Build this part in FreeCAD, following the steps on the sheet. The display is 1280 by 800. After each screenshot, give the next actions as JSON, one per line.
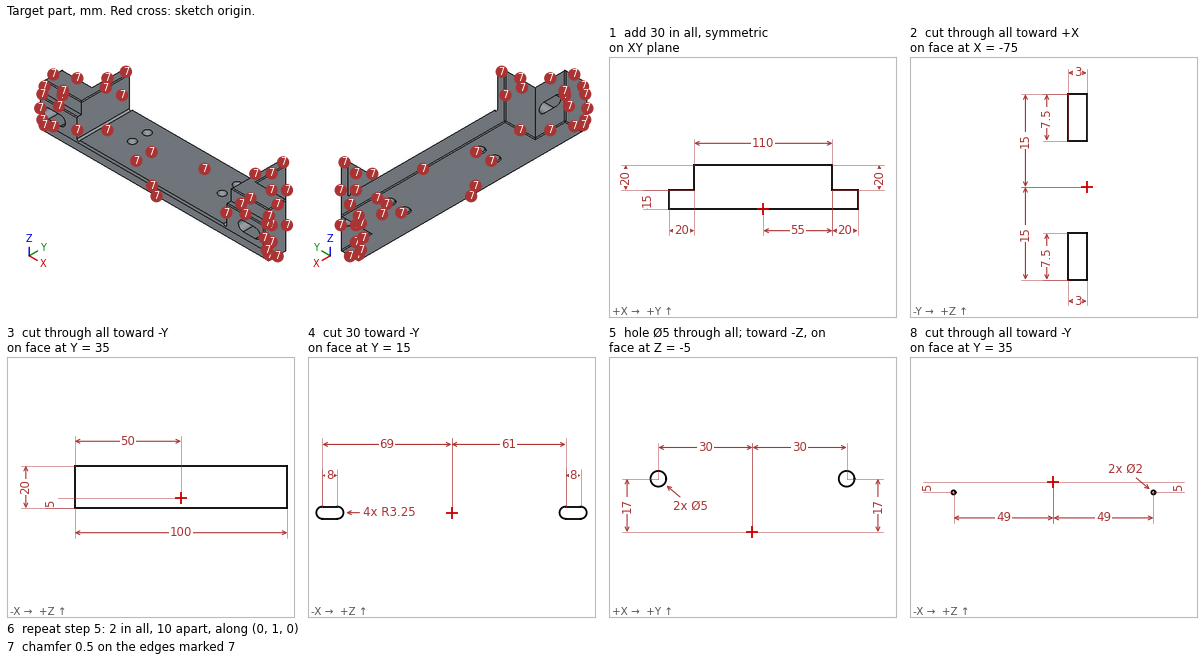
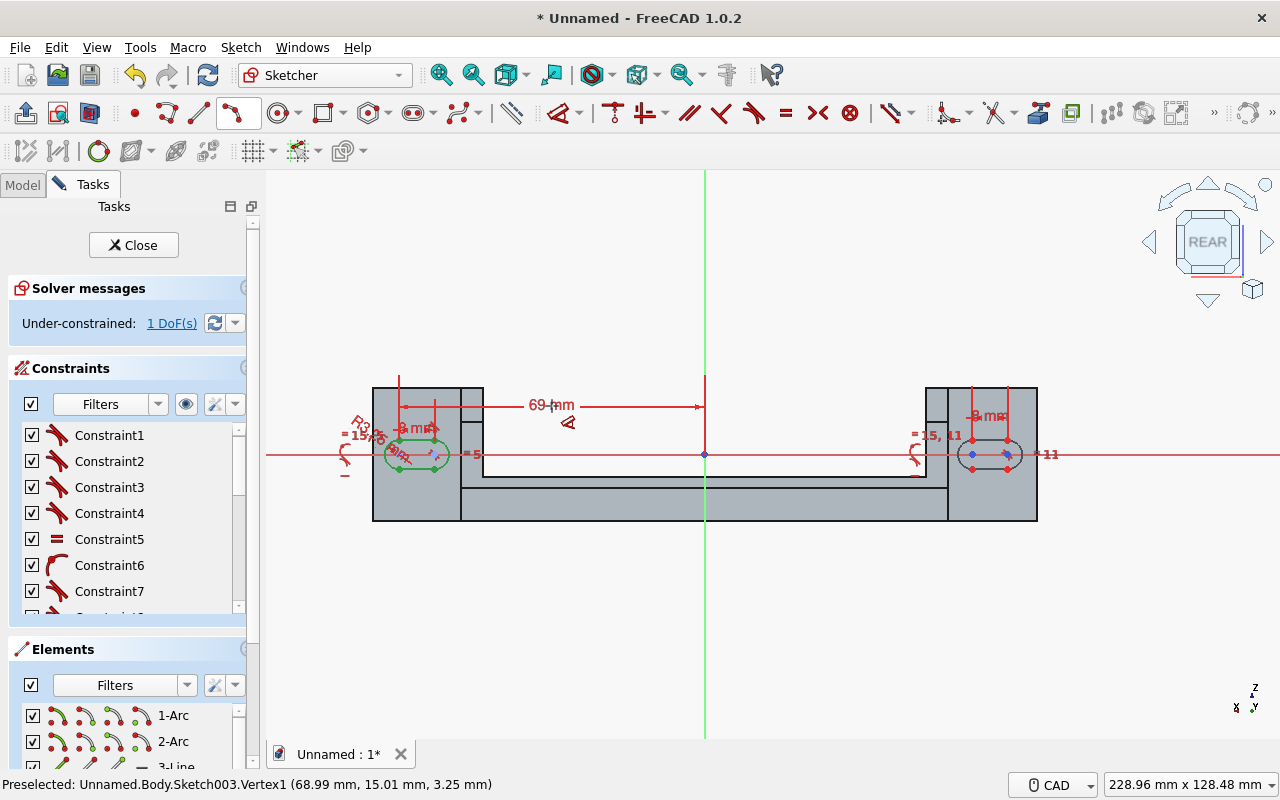
{"action": "left_click", "coordinate": [972, 440]}
{"action": "left_click", "coordinate": [839, 406]}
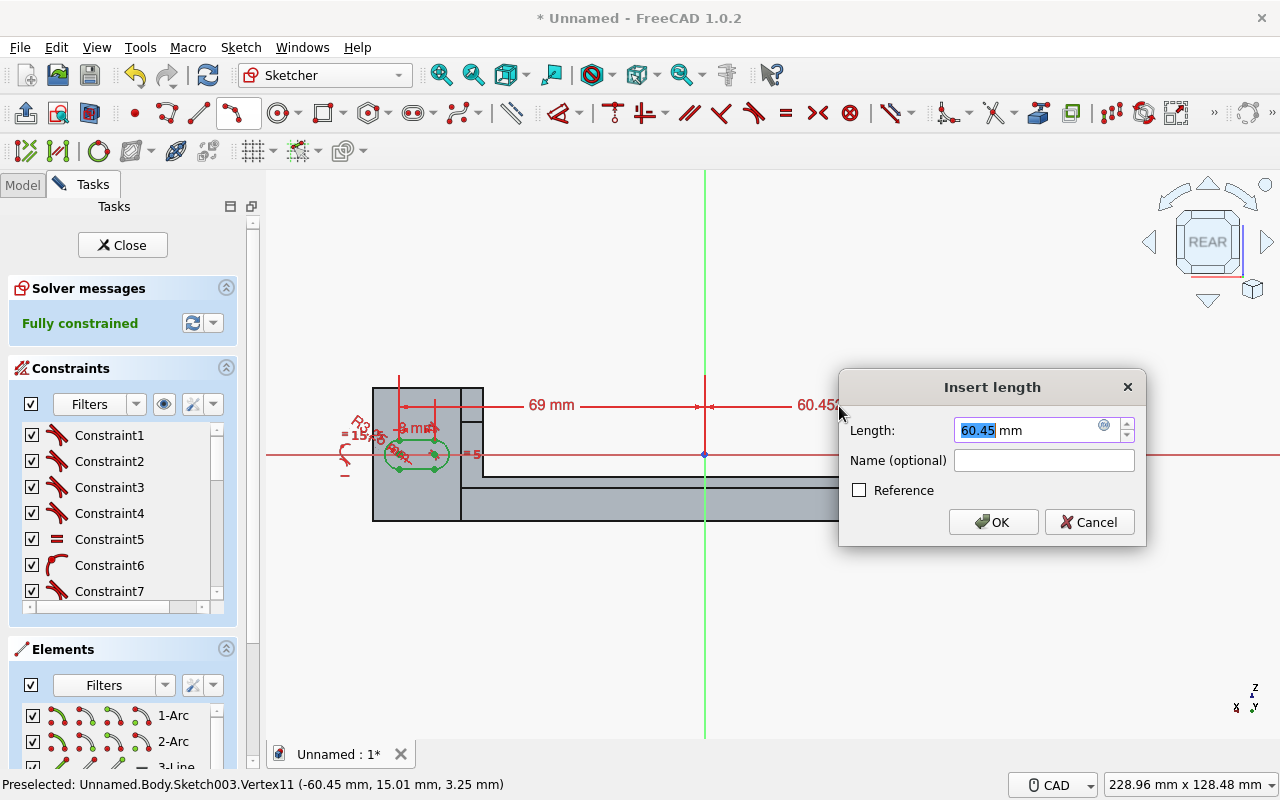
{"action": "type", "text": "61"}
{"action": "key", "text": "Return"}
{"action": "key", "text": "Escape"}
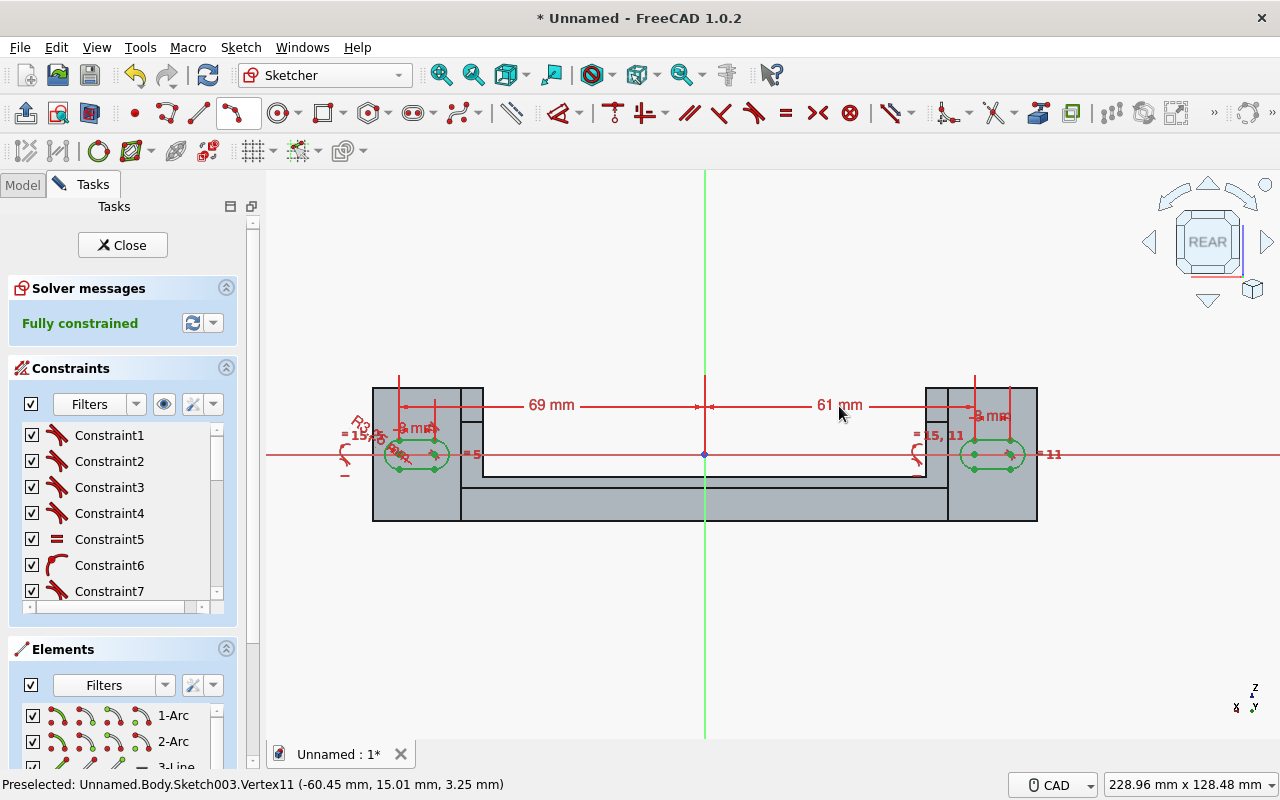
{"action": "left_click", "coordinate": [123, 245]}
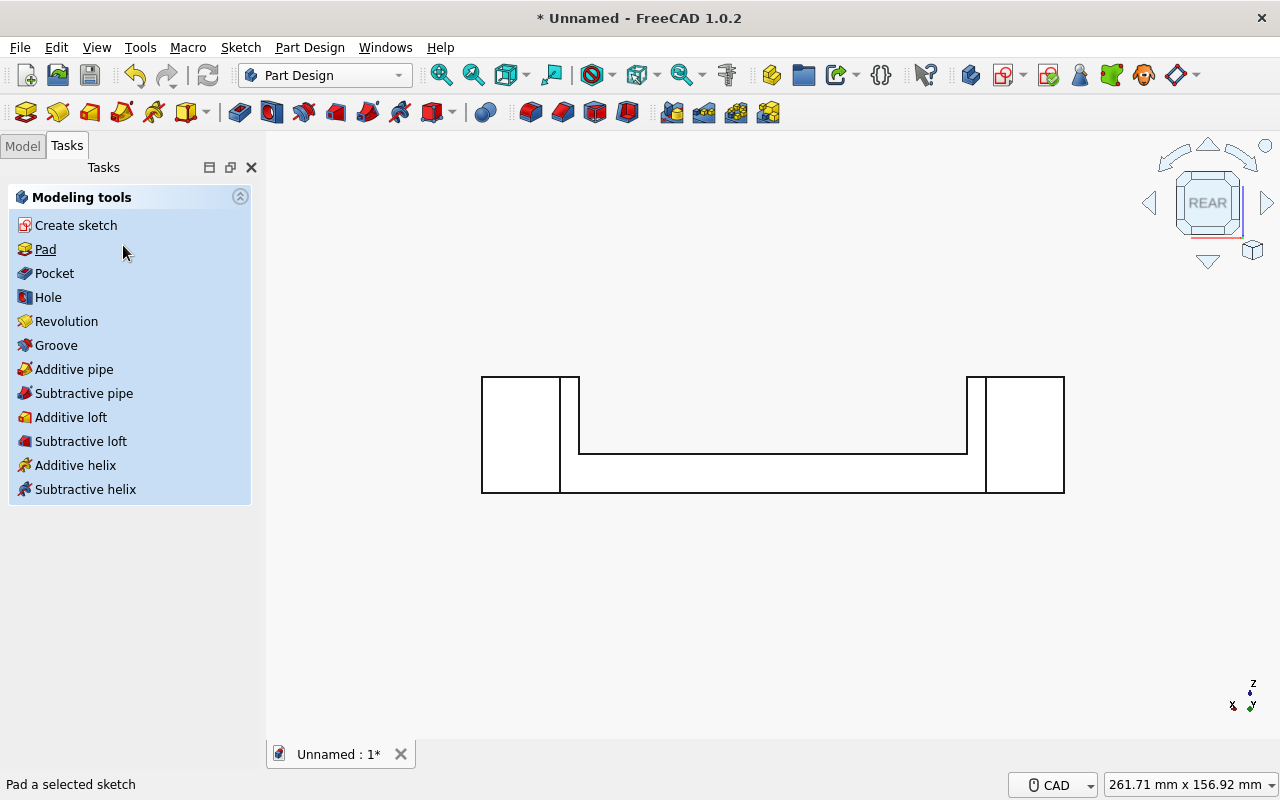
{"action": "left_click", "coordinate": [240, 112]}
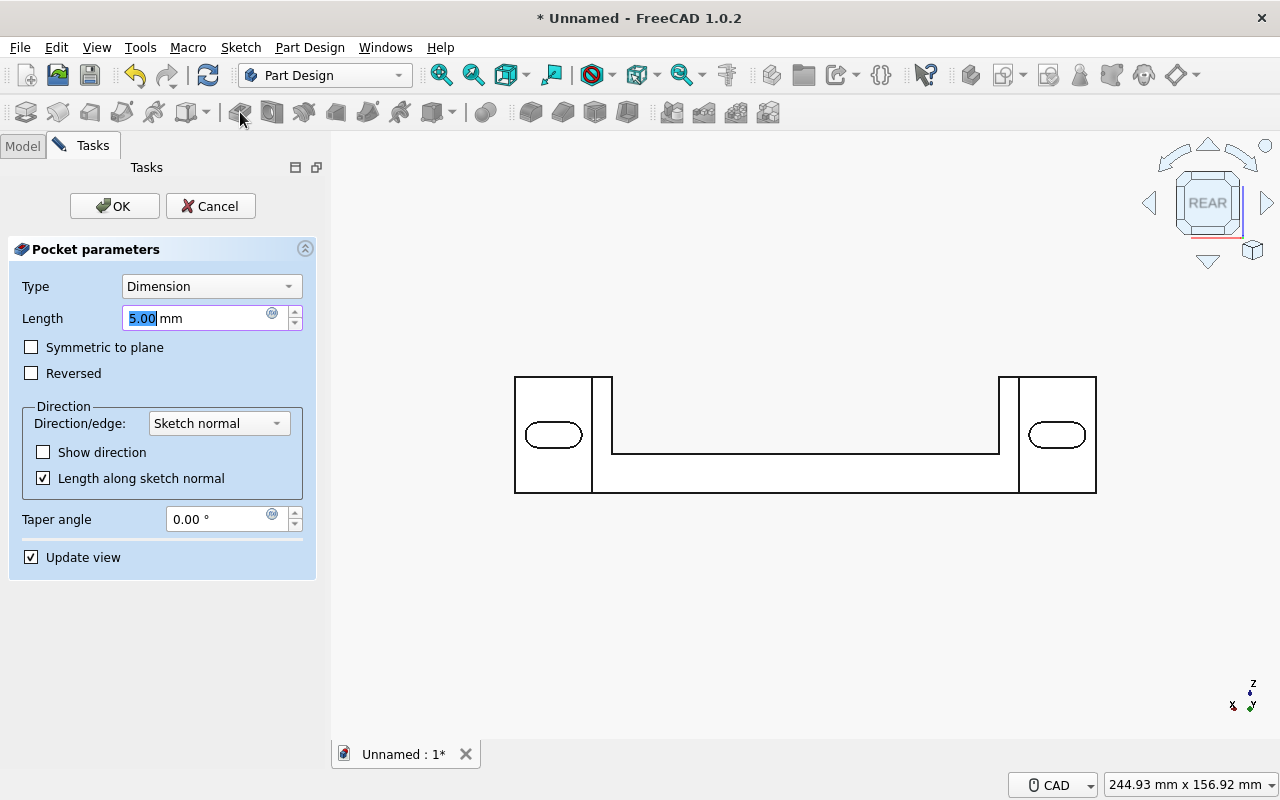
{"action": "type", "text": "30"}
{"action": "key", "text": "Tab"}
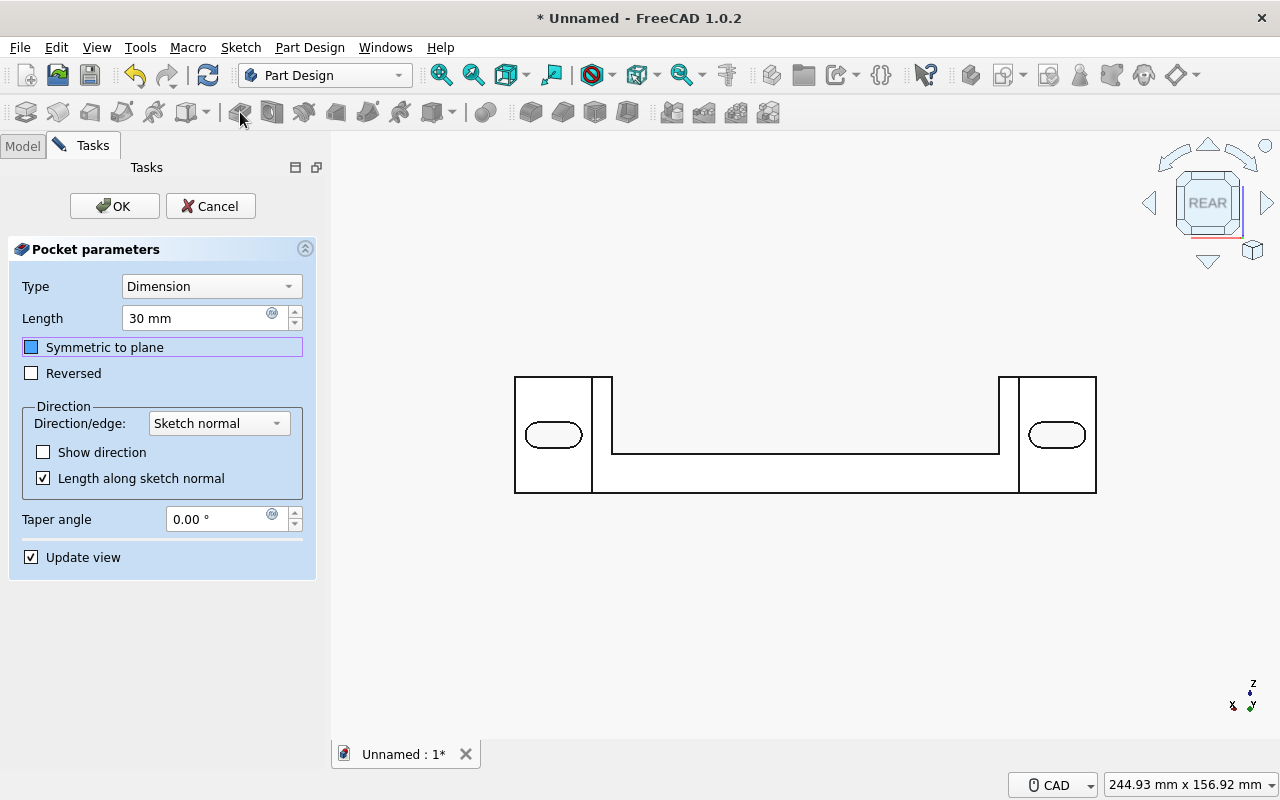
{"action": "left_click", "coordinate": [115, 206]}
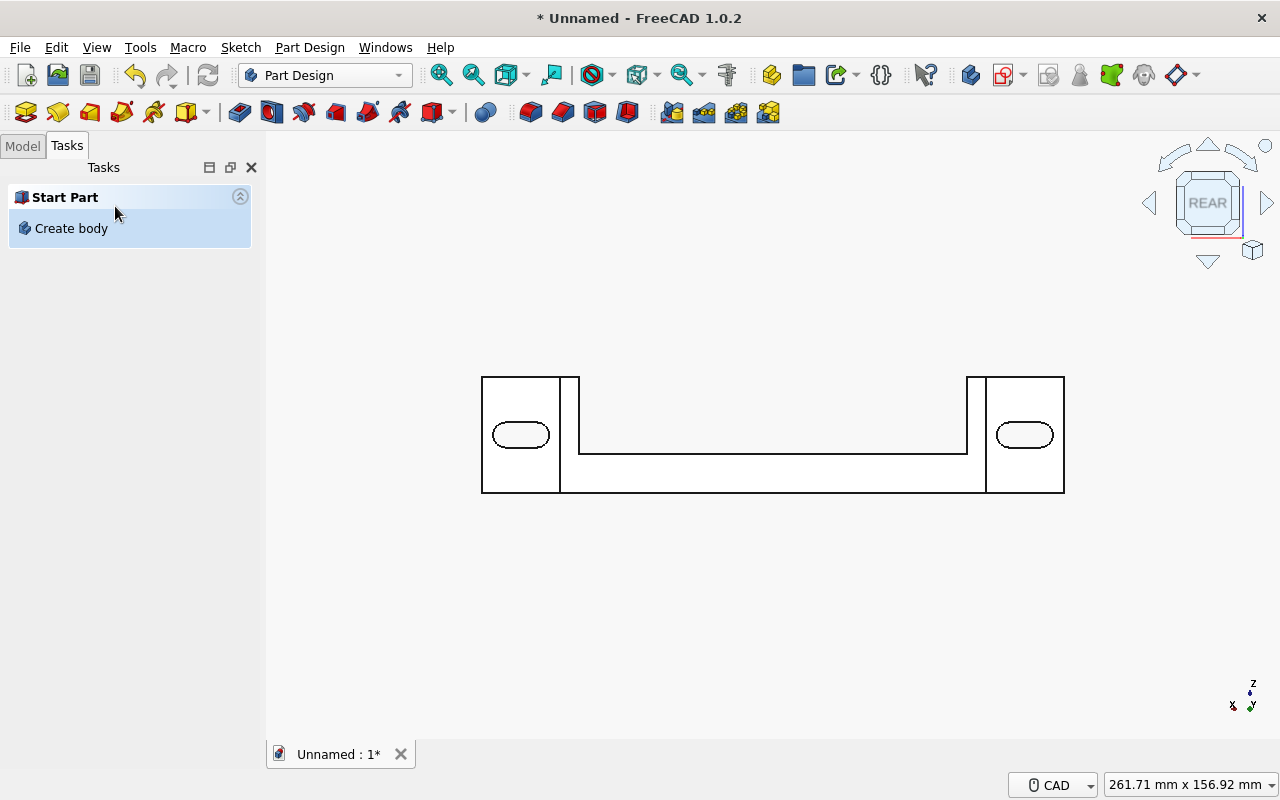
{"action": "key", "text": "0"}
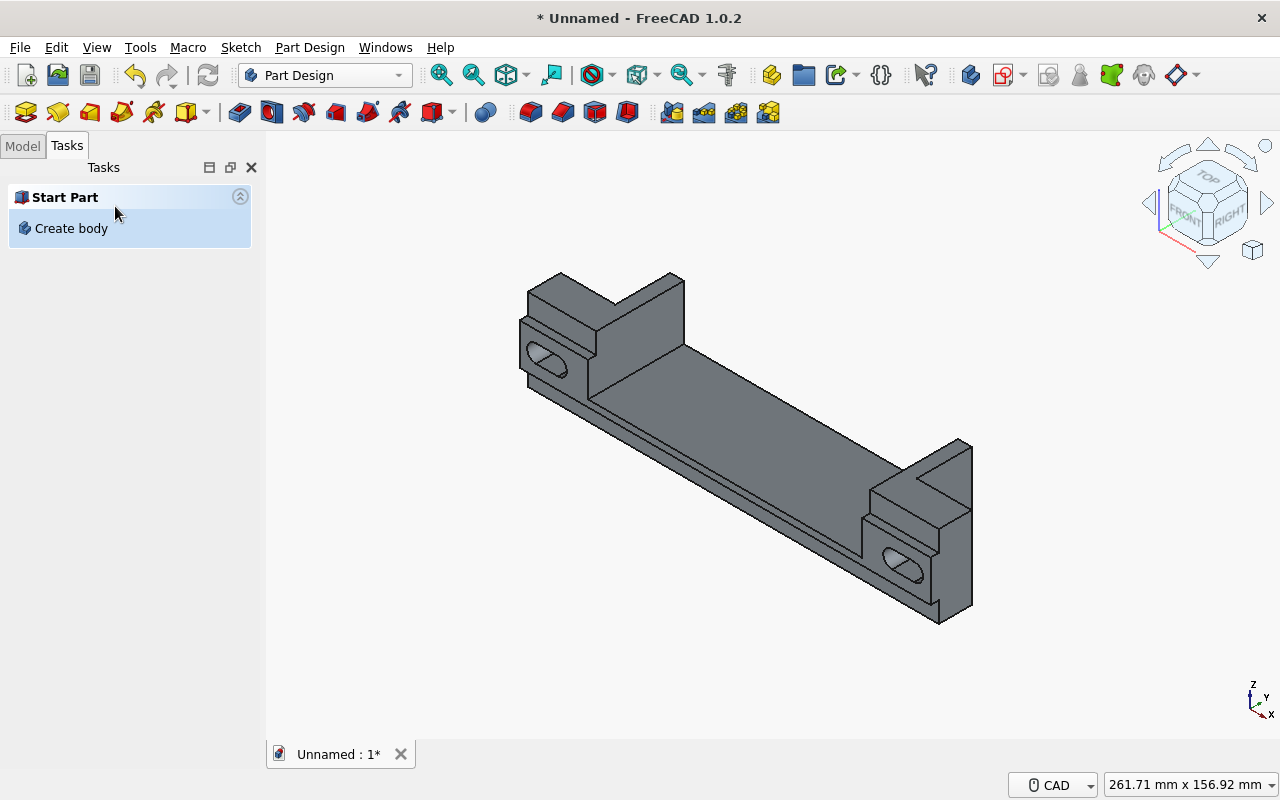
{"action": "left_click", "coordinate": [851, 495]}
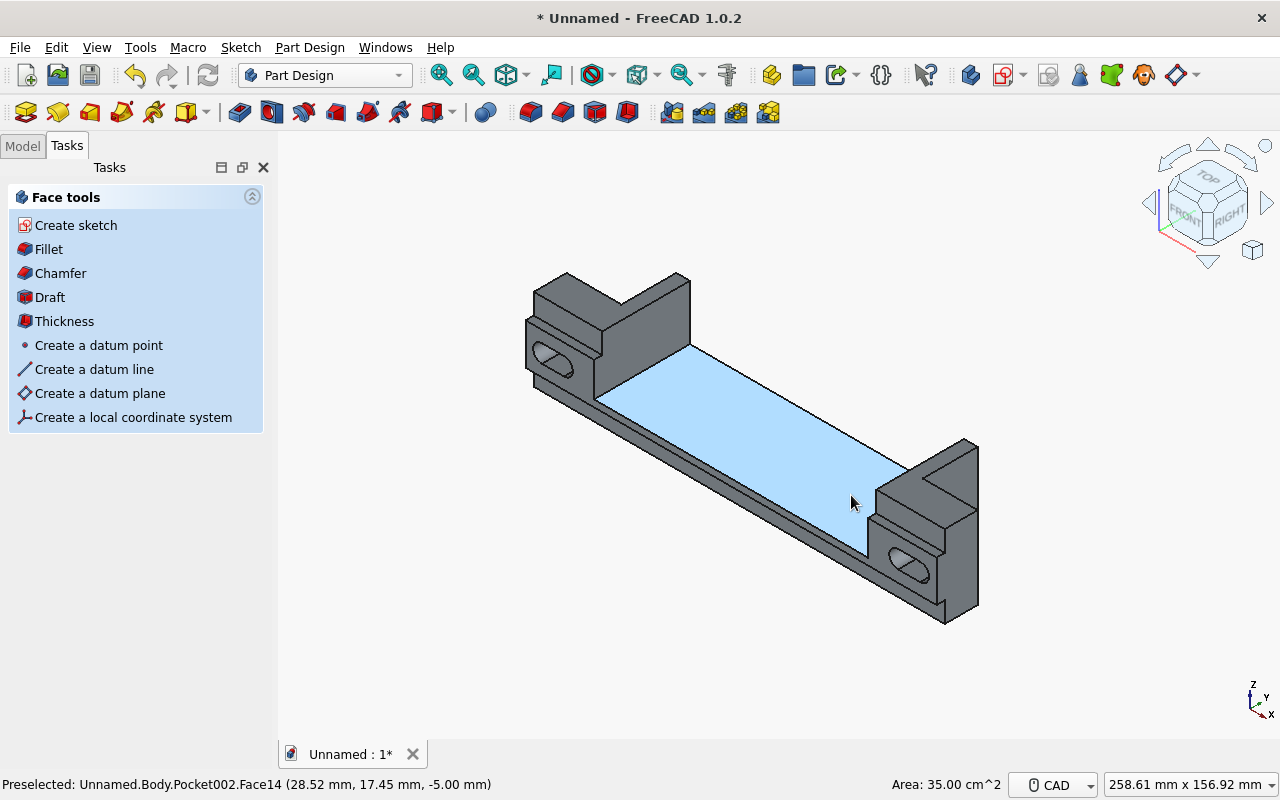
{"action": "left_click", "coordinate": [1004, 76]}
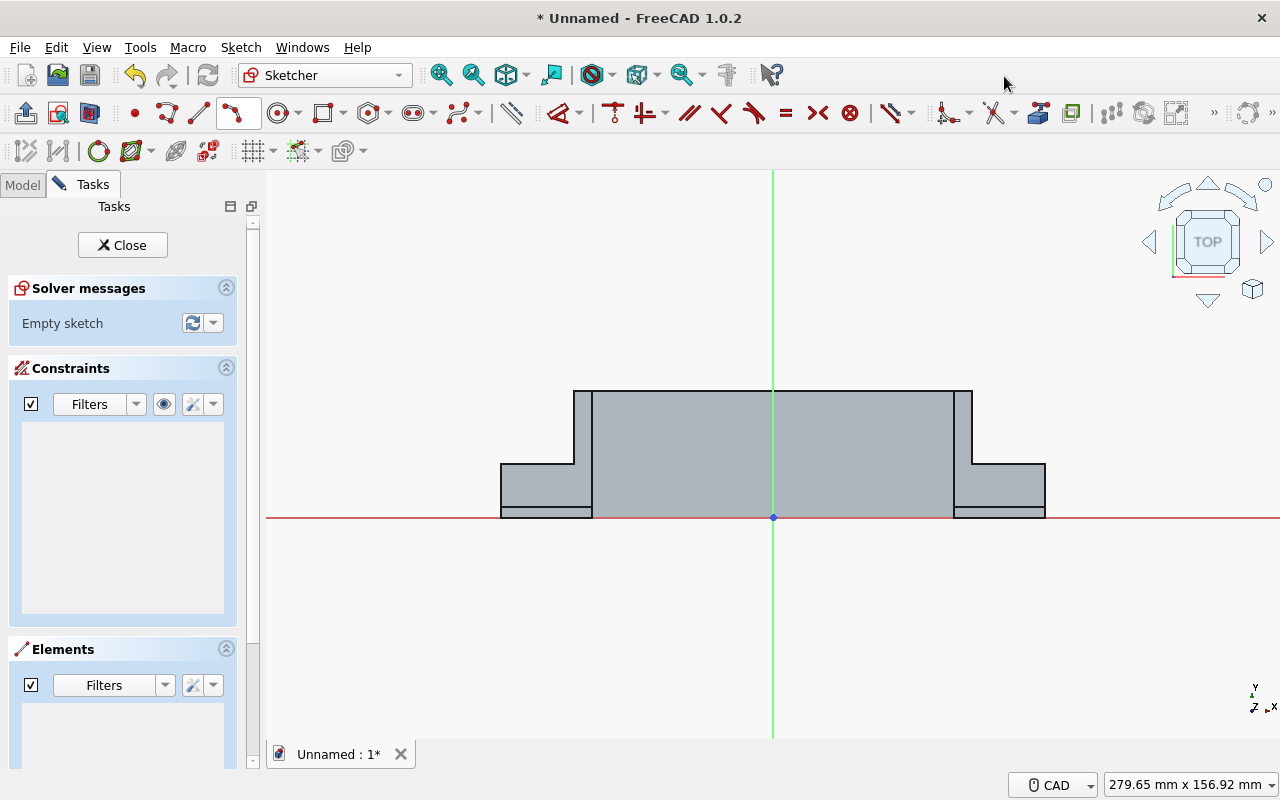
{"action": "scroll", "coordinate": [829, 506], "scroll_direction": "up", "scroll_amount": 4}